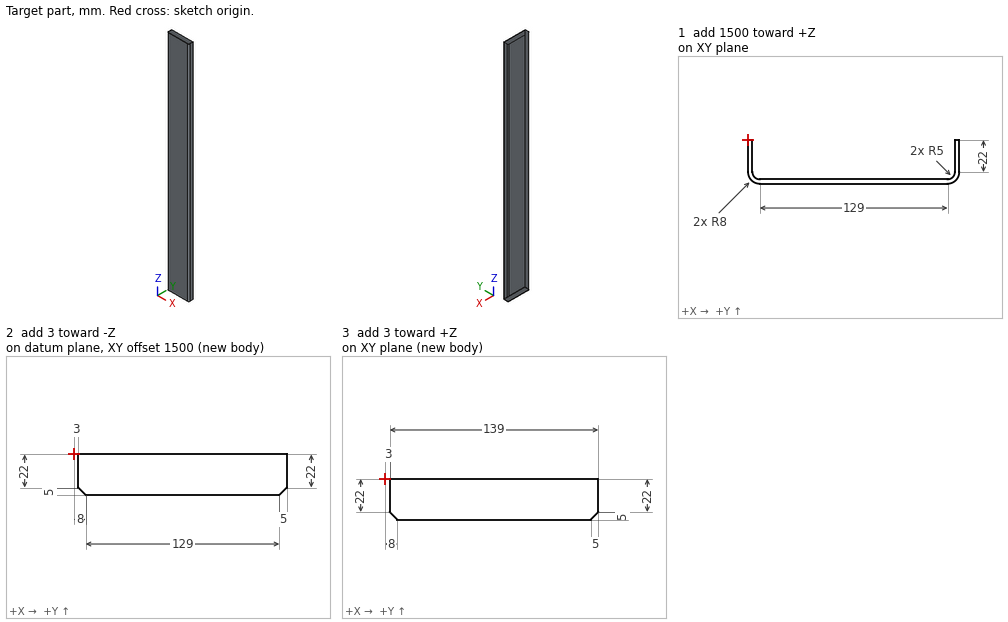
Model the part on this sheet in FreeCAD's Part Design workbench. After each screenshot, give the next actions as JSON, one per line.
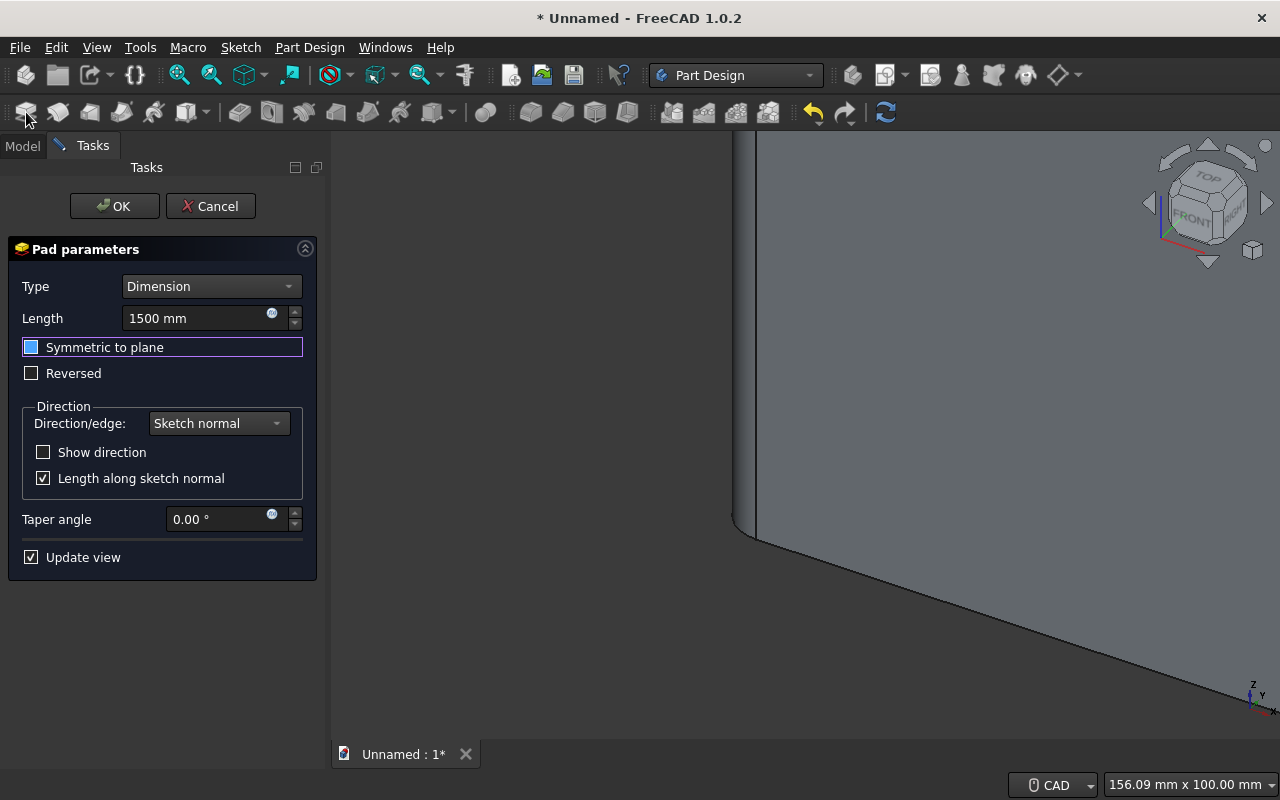
{"action": "left_click", "coordinate": [115, 206]}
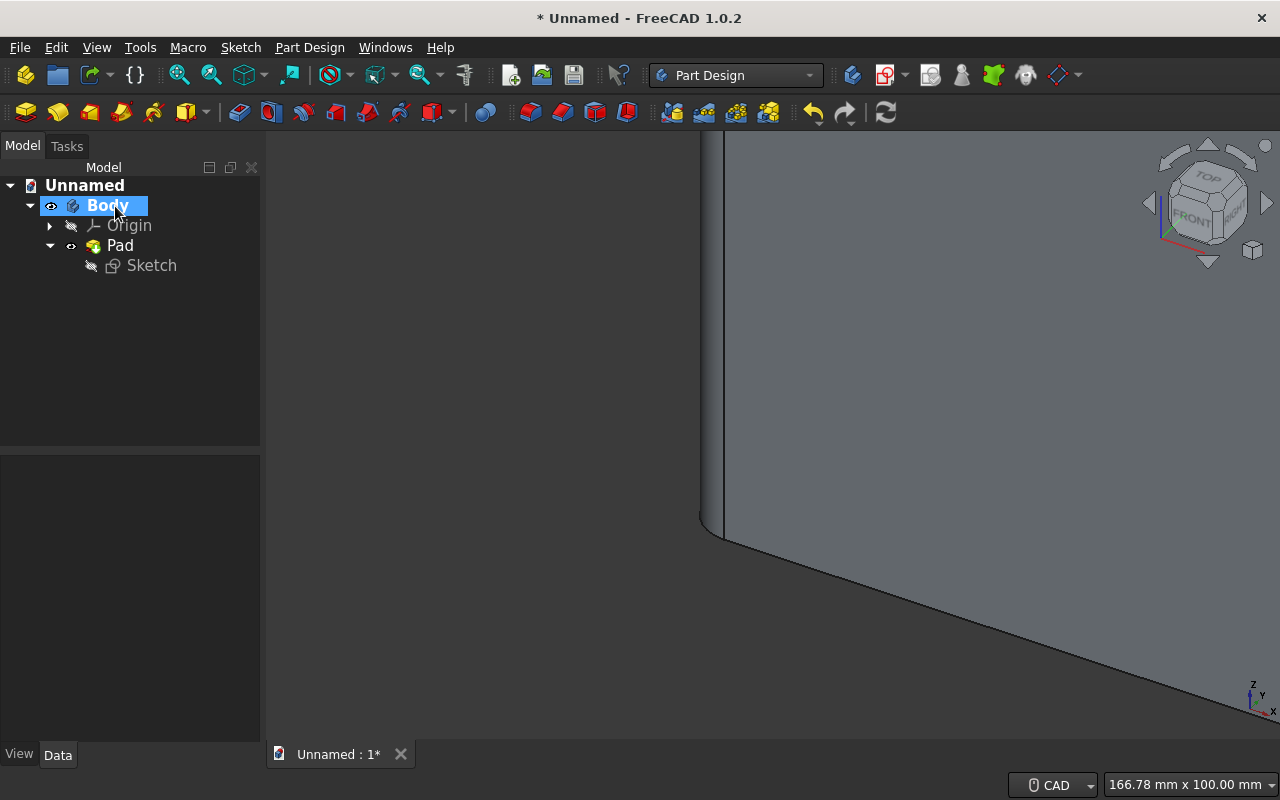
{"action": "key", "text": "v f"}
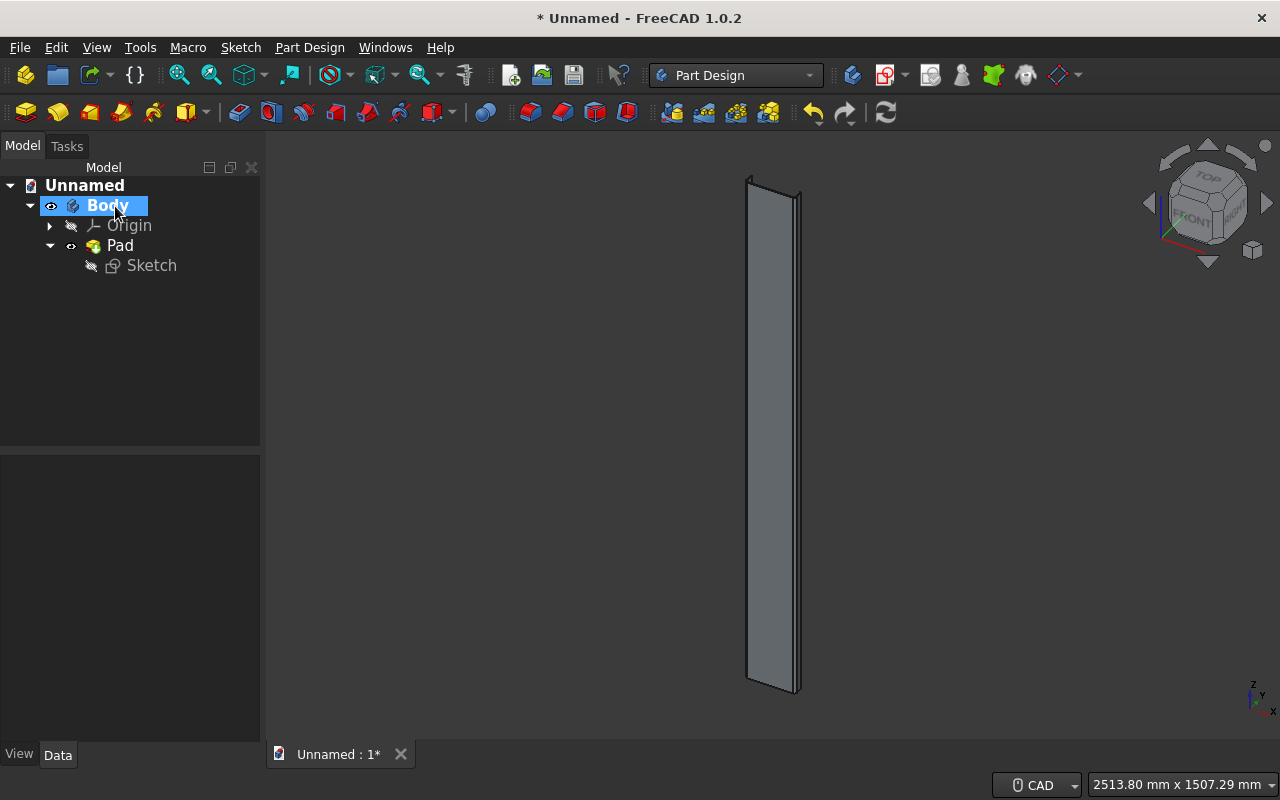
{"action": "left_click", "coordinate": [854, 76]}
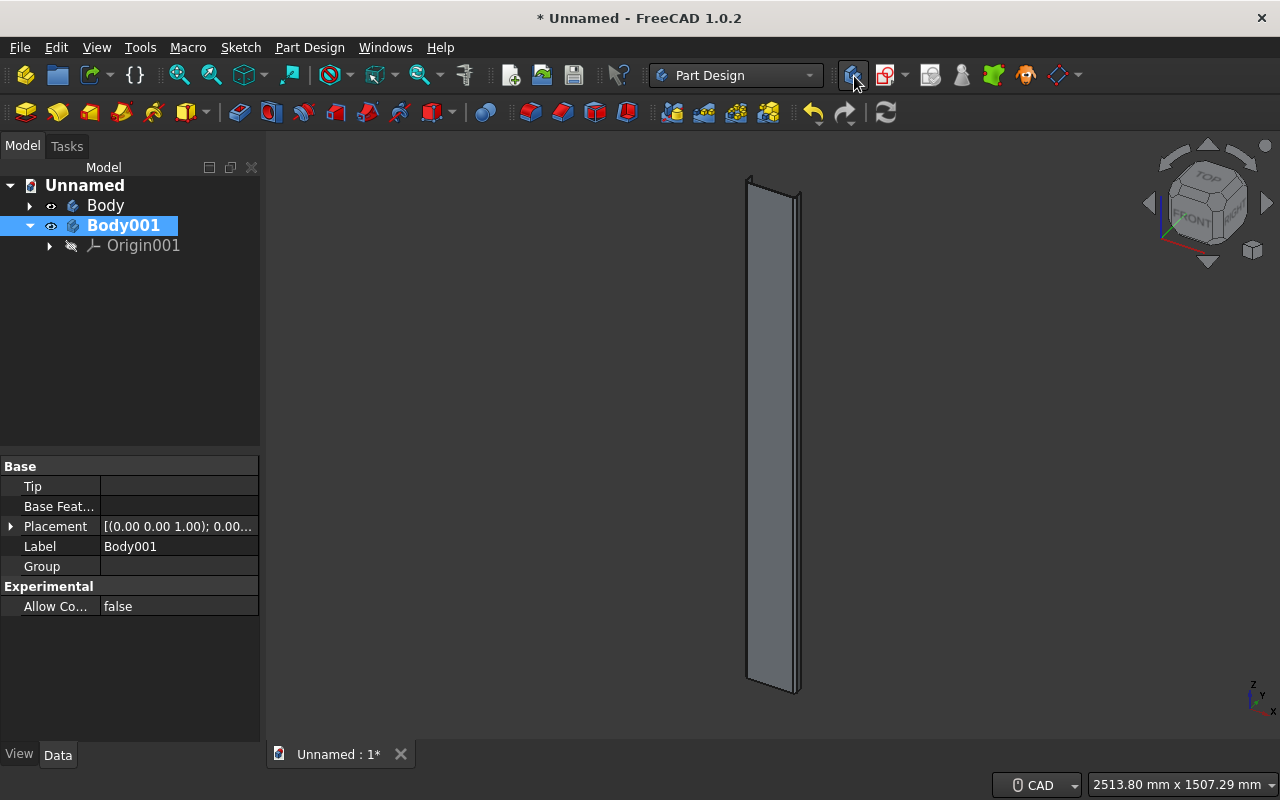
{"action": "left_click", "coordinate": [50, 246]}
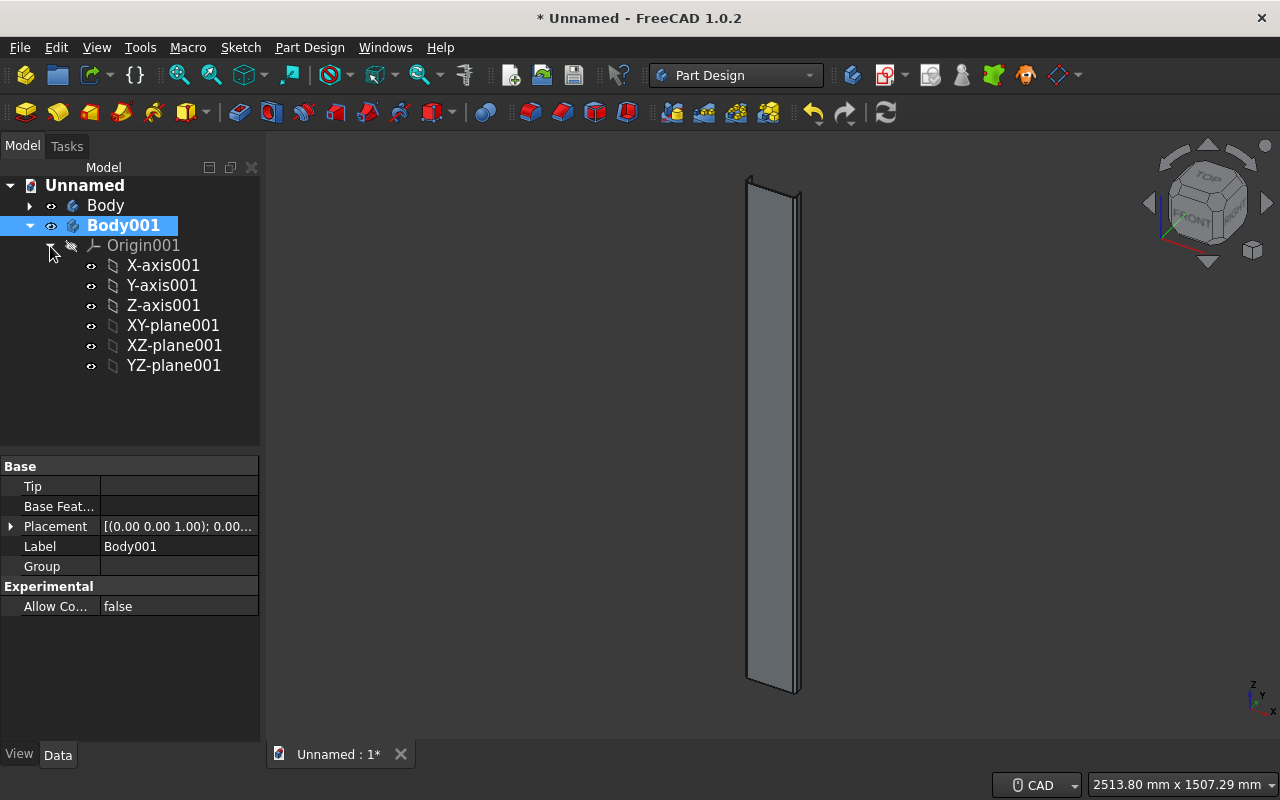
{"action": "left_click", "coordinate": [136, 326]}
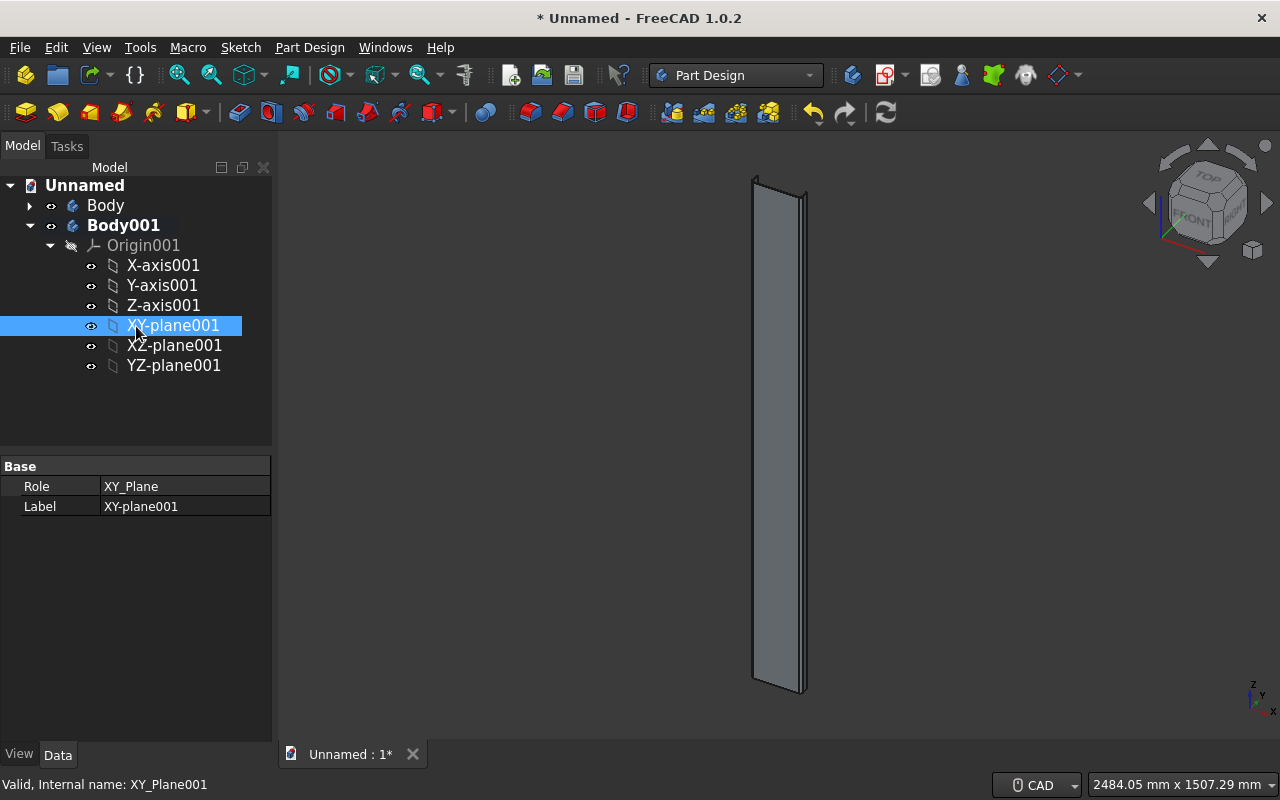
{"action": "left_click", "coordinate": [1058, 76]}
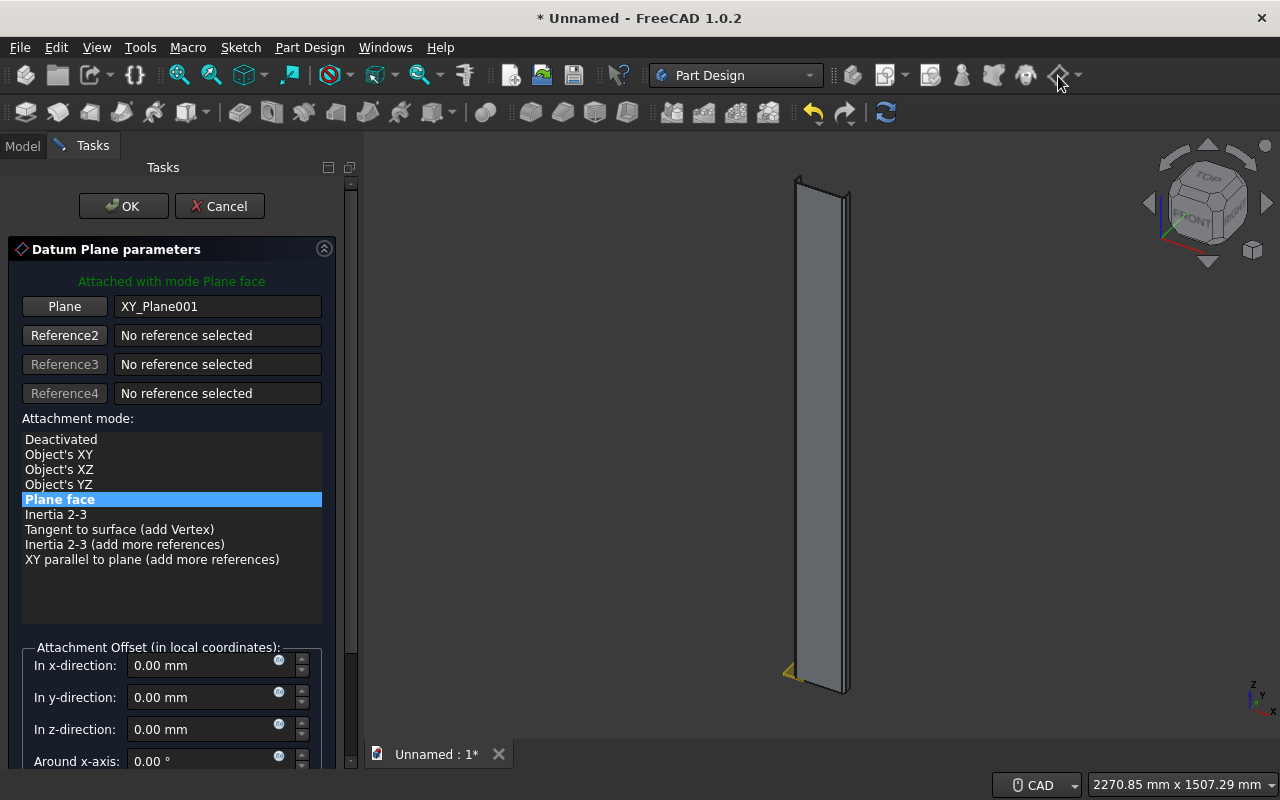
{"action": "triple_click", "coordinate": [210, 729]}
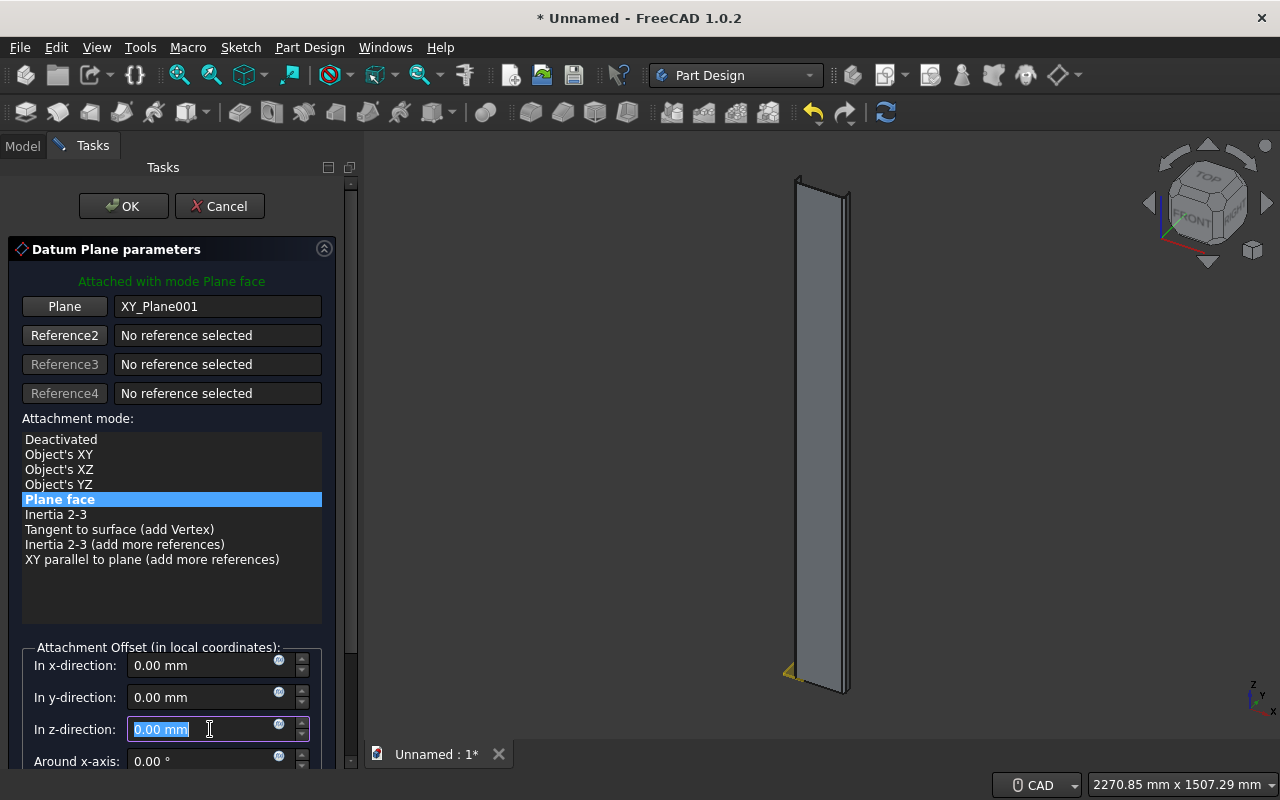
{"action": "type", "text": "1500"}
{"action": "key", "text": "Tab"}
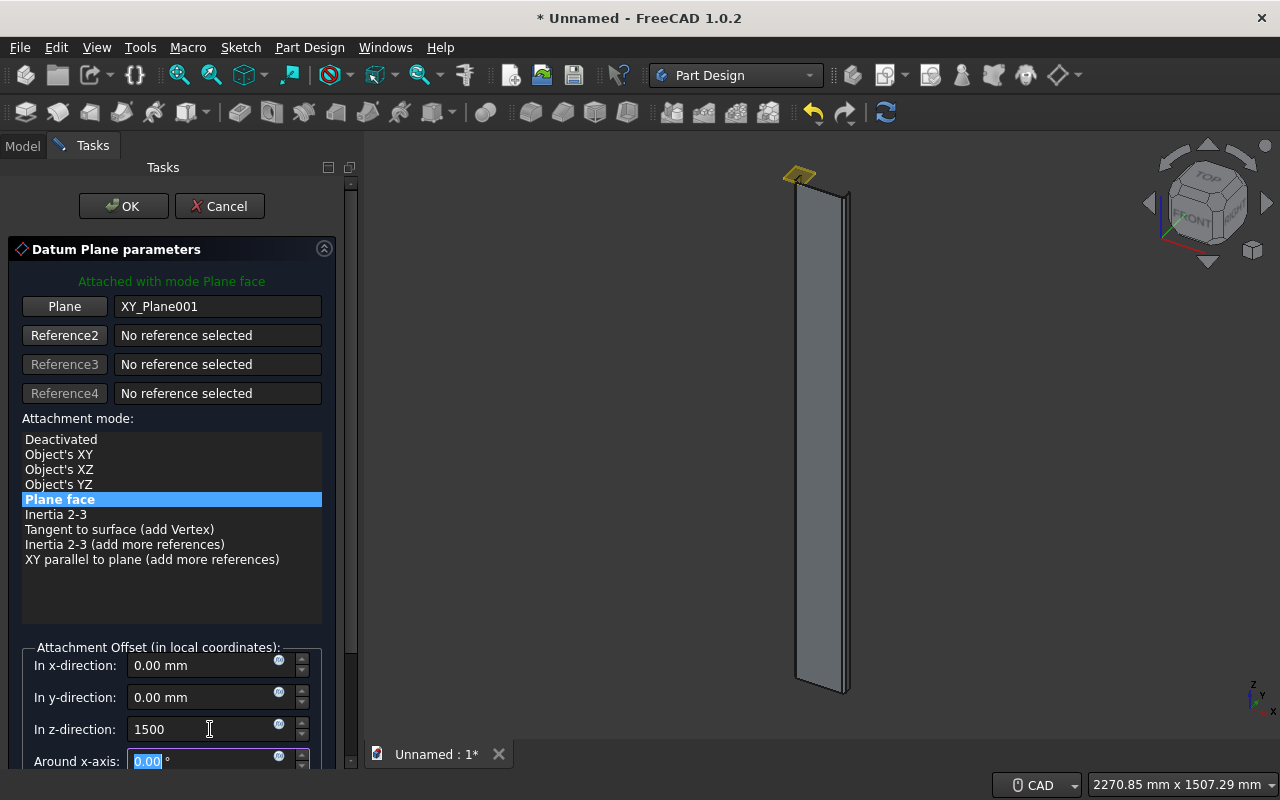
{"action": "left_click", "coordinate": [124, 206]}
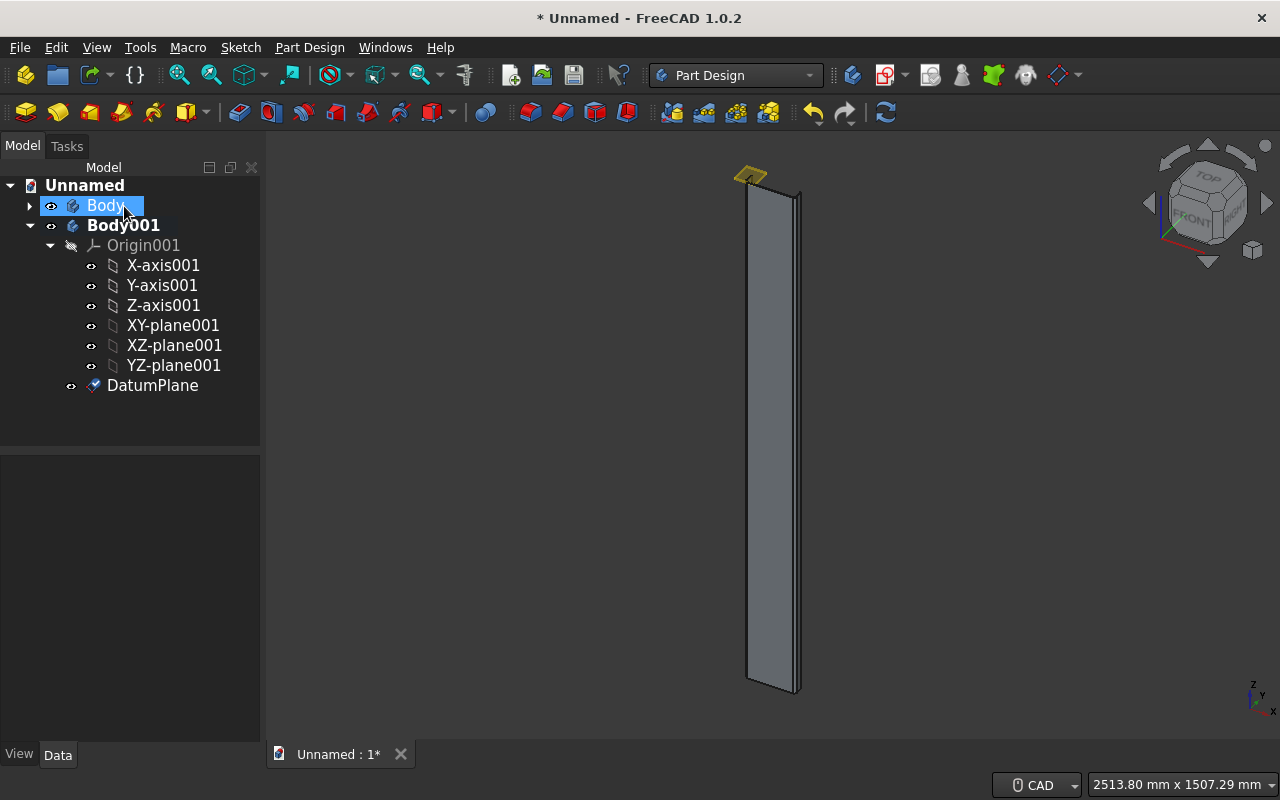
{"action": "left_click", "coordinate": [116, 386]}